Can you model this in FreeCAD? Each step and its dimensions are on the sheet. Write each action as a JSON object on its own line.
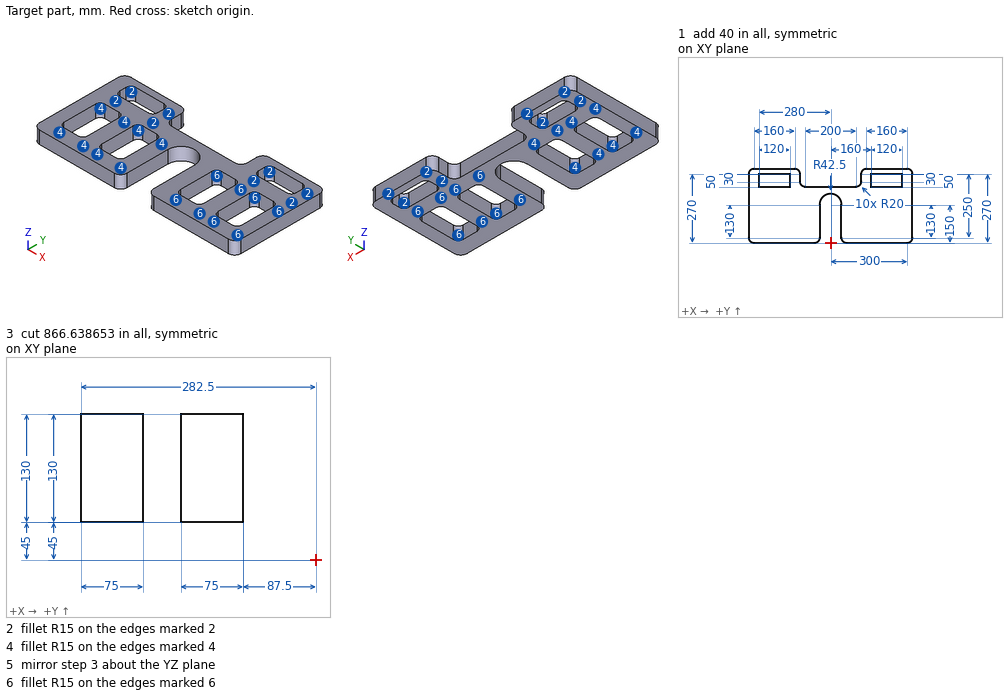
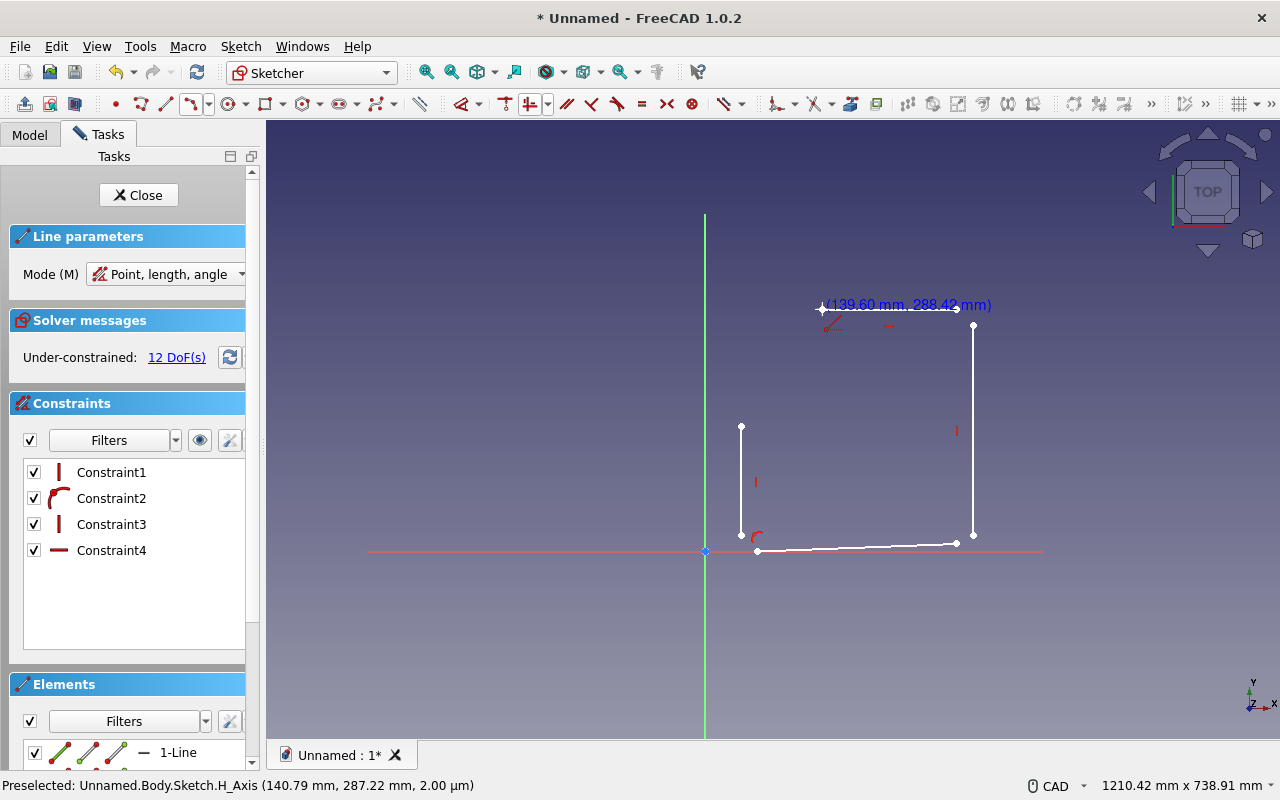
{"action": "left_click", "coordinate": [806, 325]}
{"action": "left_click", "coordinate": [806, 351]}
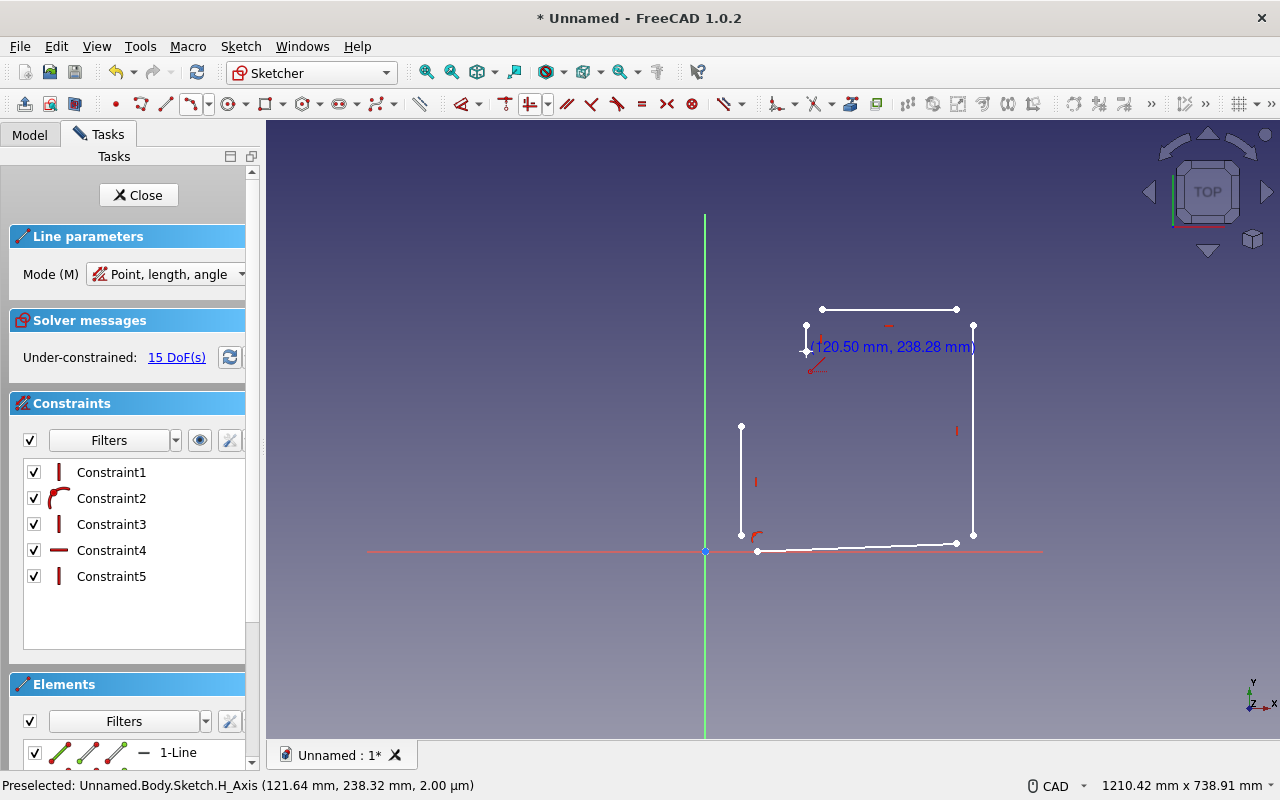
{"action": "left_click", "coordinate": [789, 367]}
{"action": "left_click", "coordinate": [621, 367]}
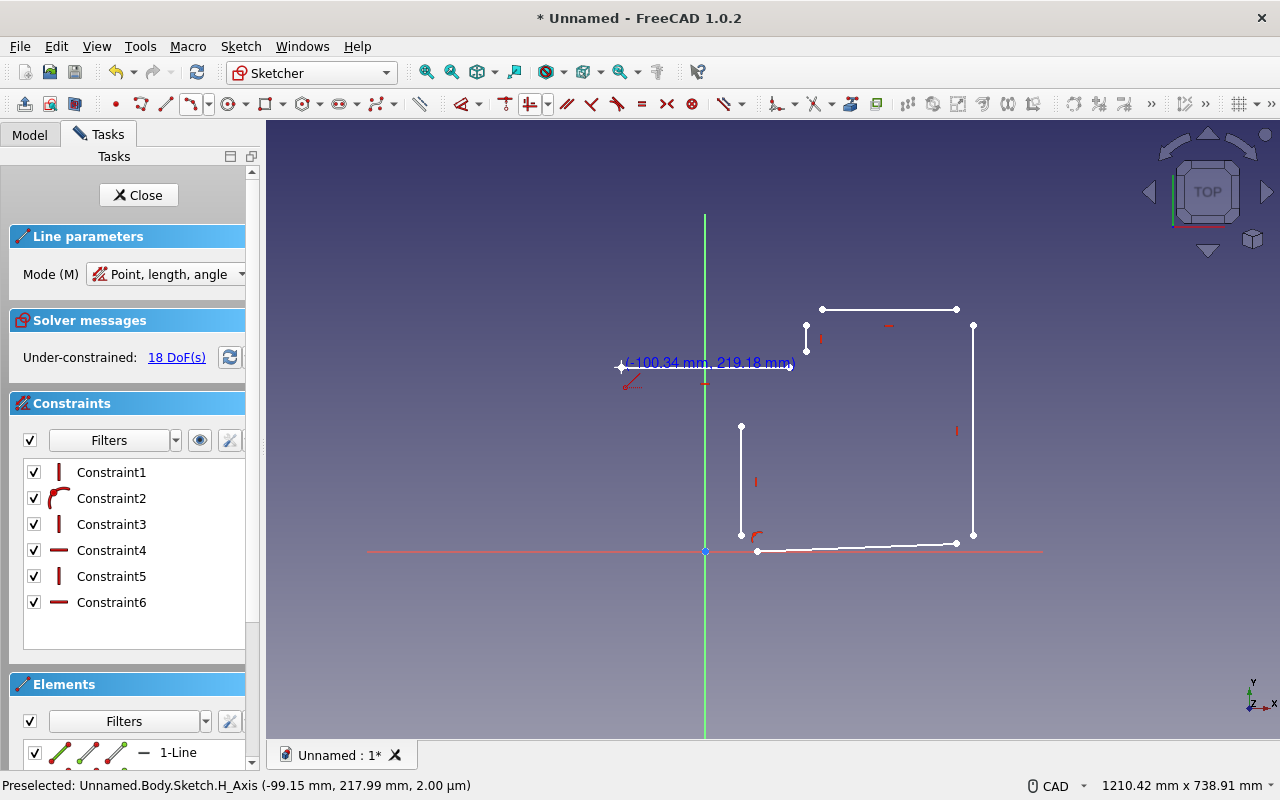
{"action": "left_click", "coordinate": [605, 351]}
{"action": "left_click", "coordinate": [605, 325]}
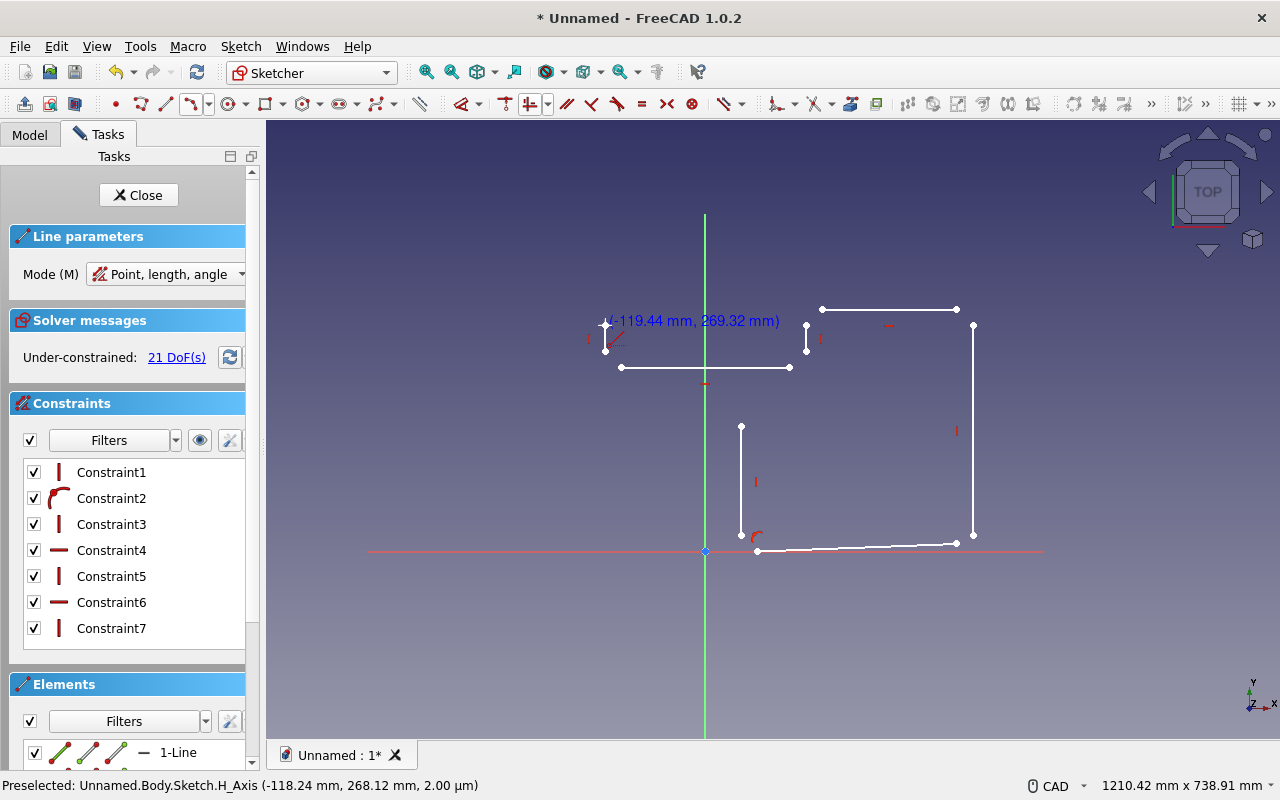
{"action": "left_click", "coordinate": [588, 309]}
{"action": "left_click", "coordinate": [454, 309]}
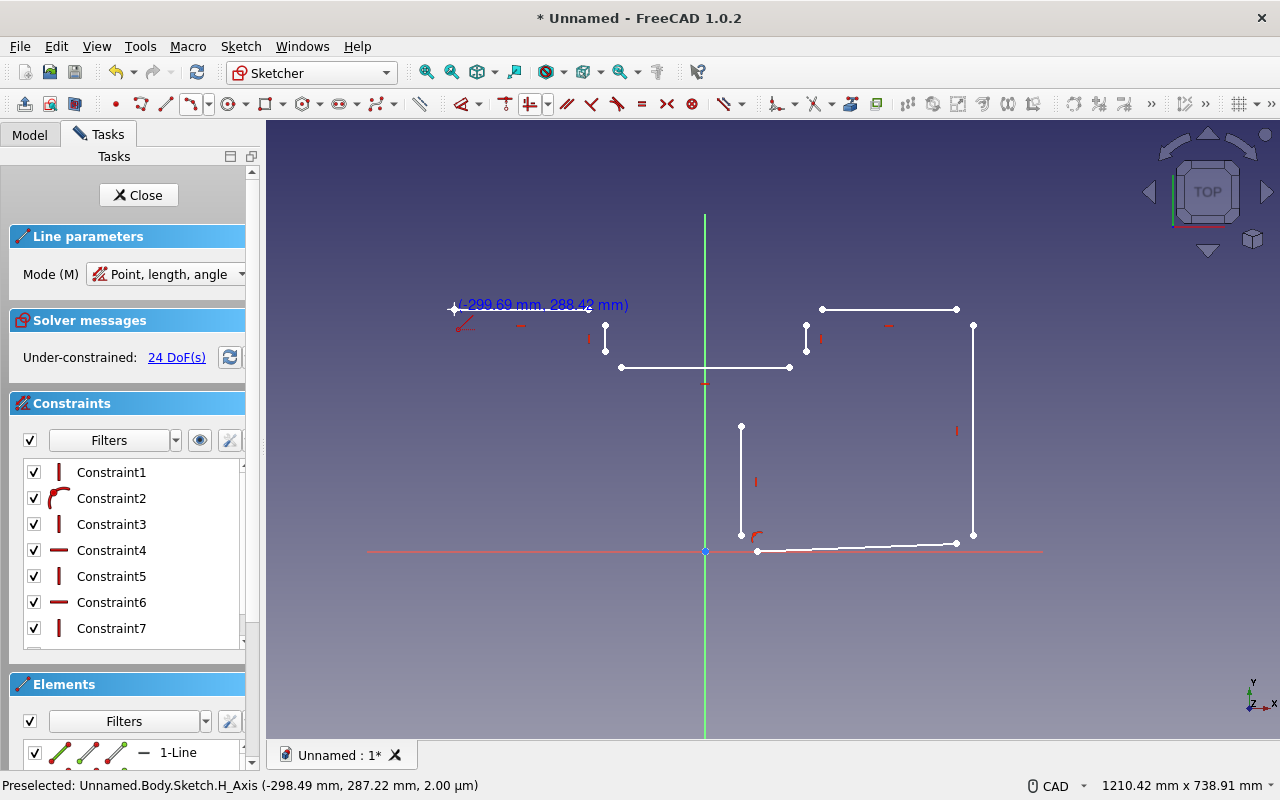
{"action": "left_click", "coordinate": [437, 325]}
{"action": "left_click", "coordinate": [437, 535]}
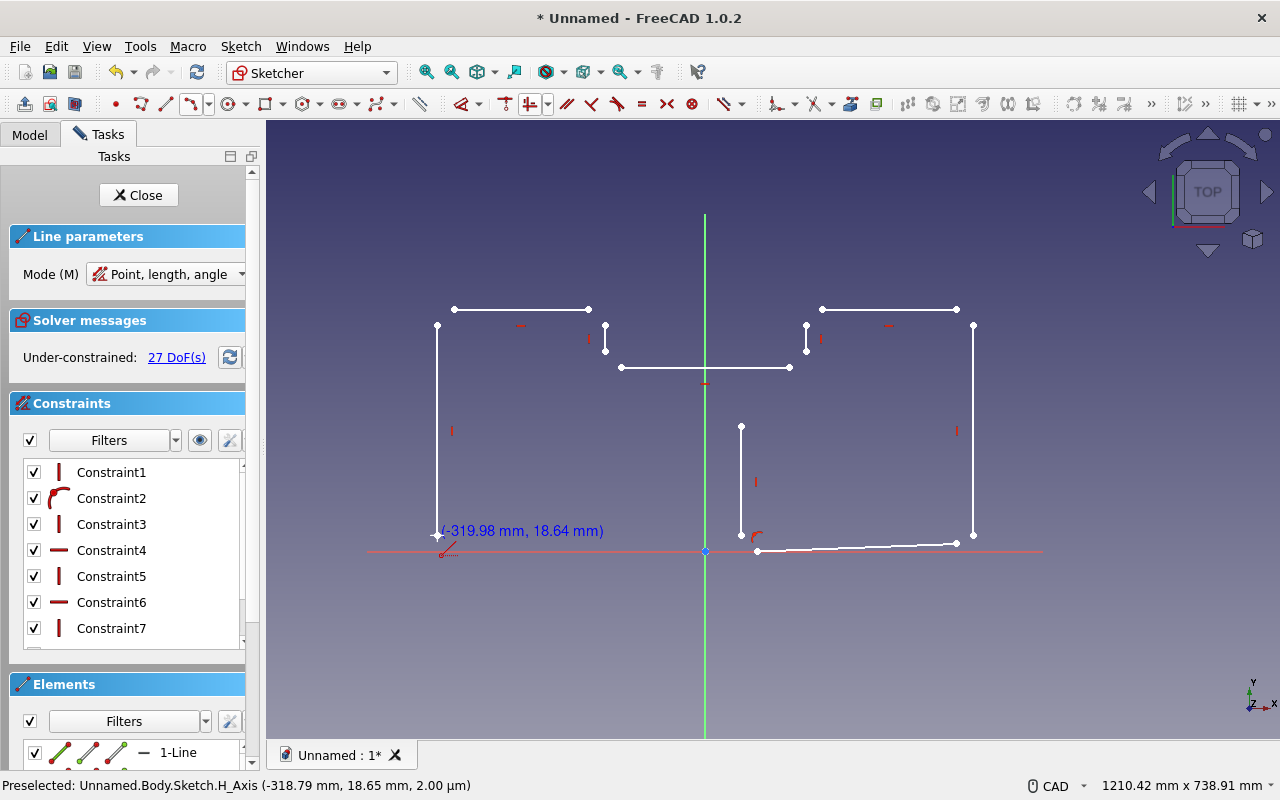
{"action": "left_click", "coordinate": [454, 552]}
{"action": "left_click", "coordinate": [653, 543]}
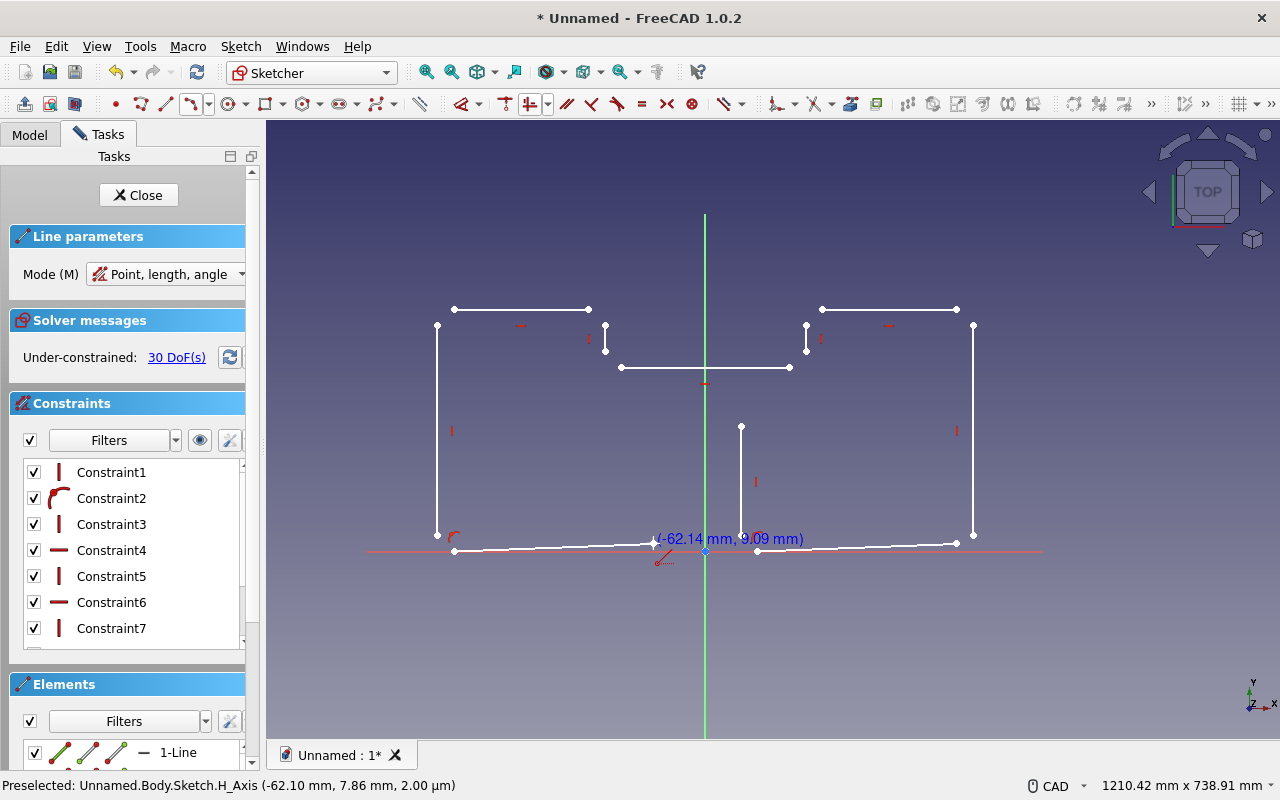
{"action": "left_click", "coordinate": [669, 535]}
{"action": "left_click", "coordinate": [669, 426]}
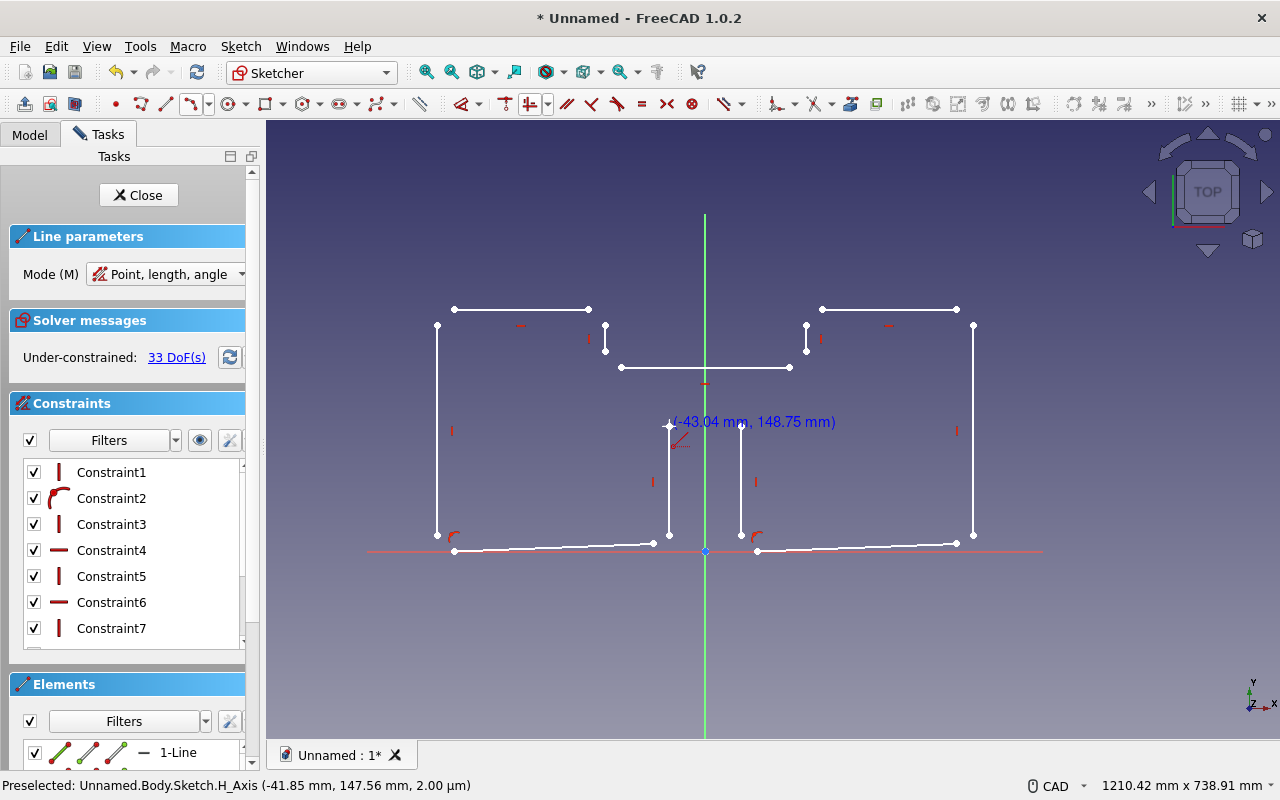
{"action": "key", "text": "g 3 a"}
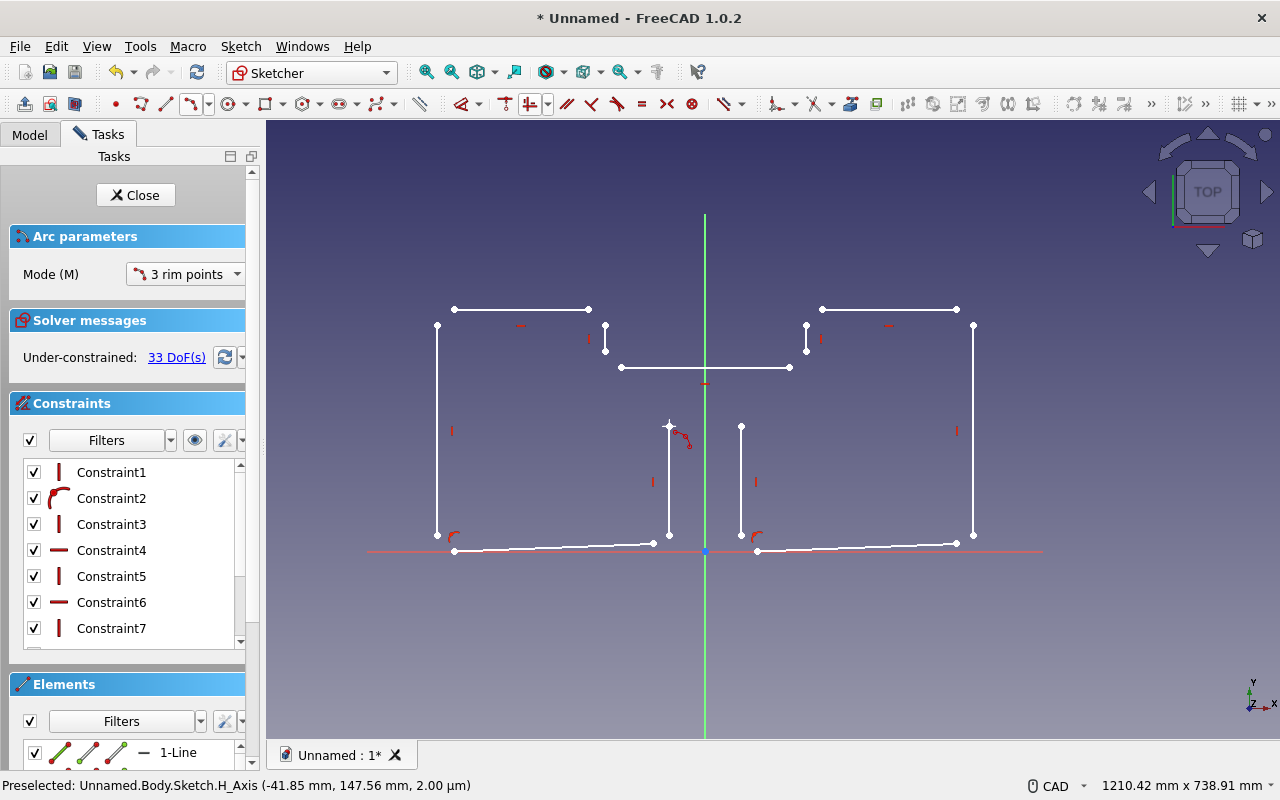
{"action": "left_click", "coordinate": [741, 536]}
{"action": "left_click", "coordinate": [757, 552]}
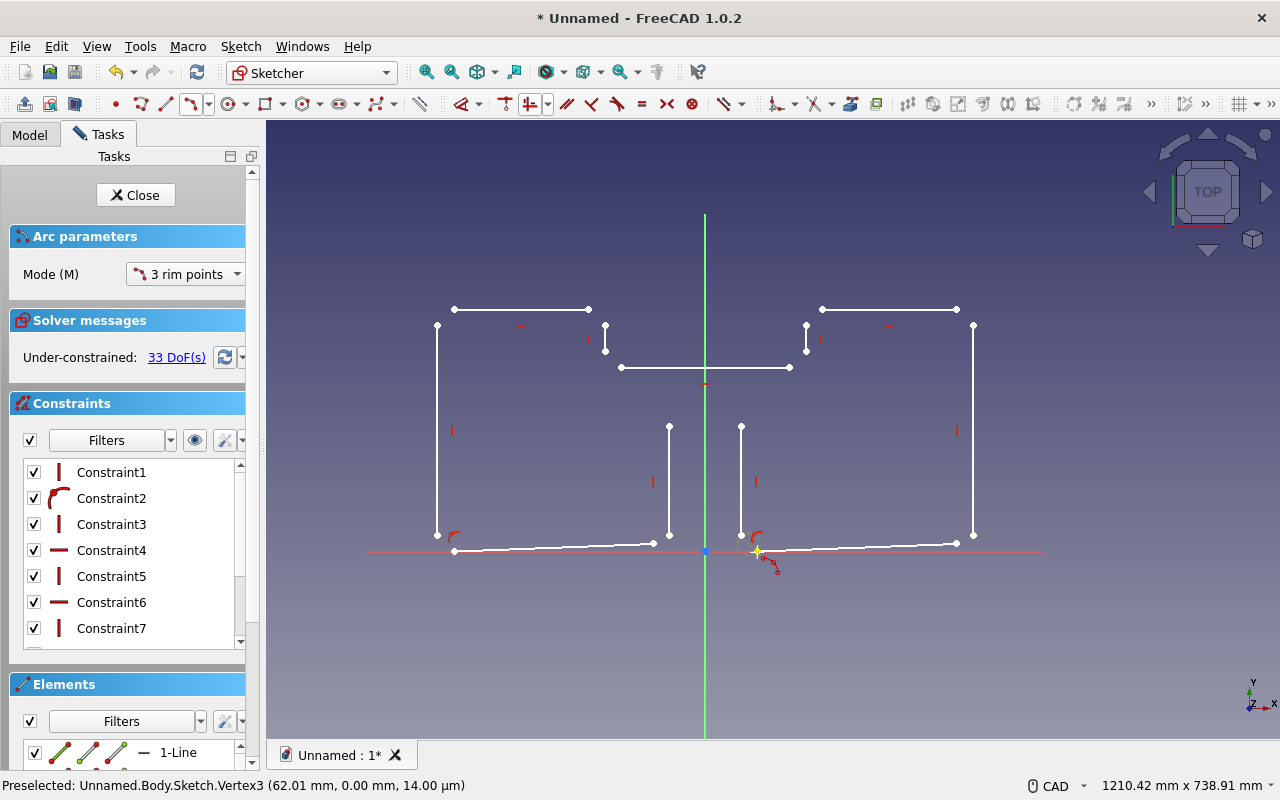
{"action": "scroll", "coordinate": [746, 547], "scroll_direction": "up", "scroll_amount": 6}